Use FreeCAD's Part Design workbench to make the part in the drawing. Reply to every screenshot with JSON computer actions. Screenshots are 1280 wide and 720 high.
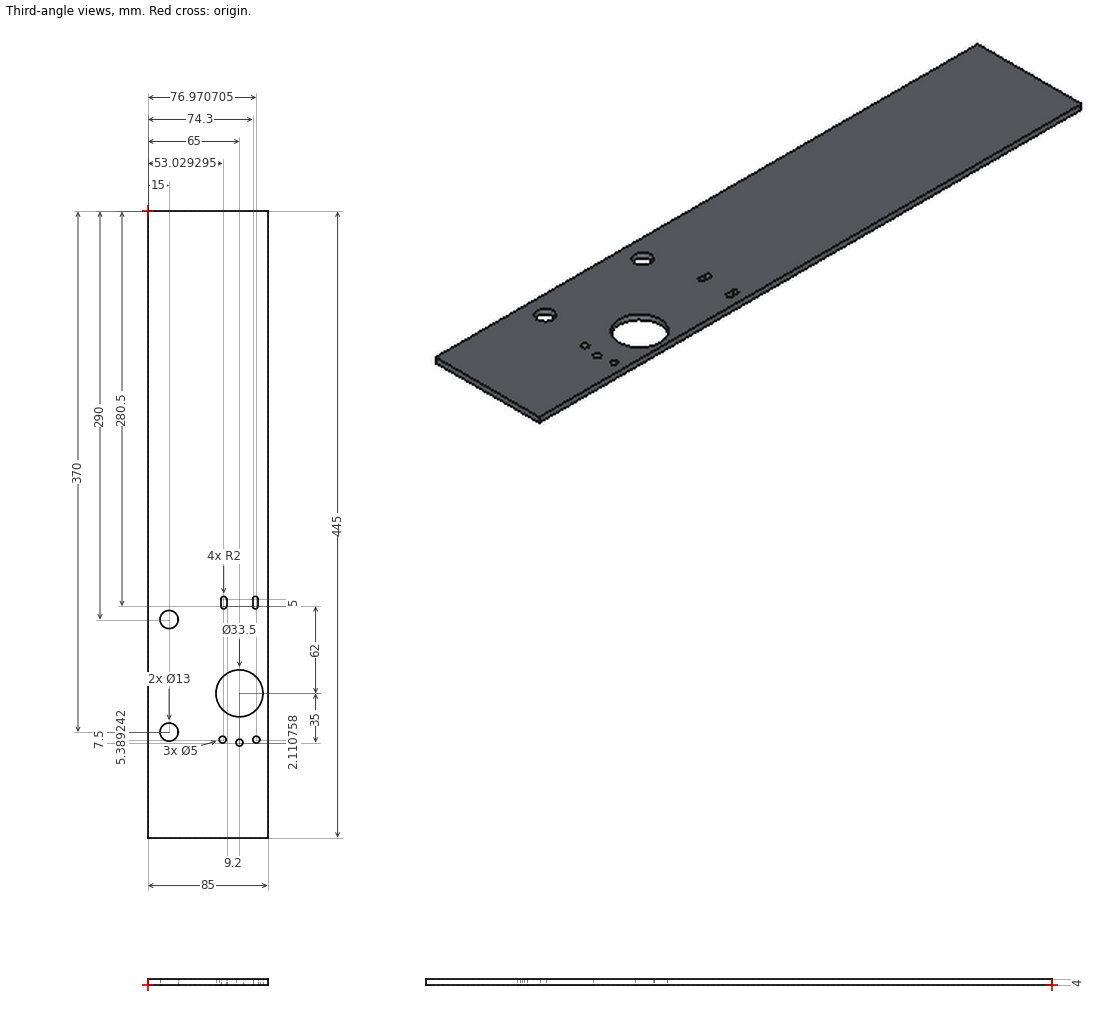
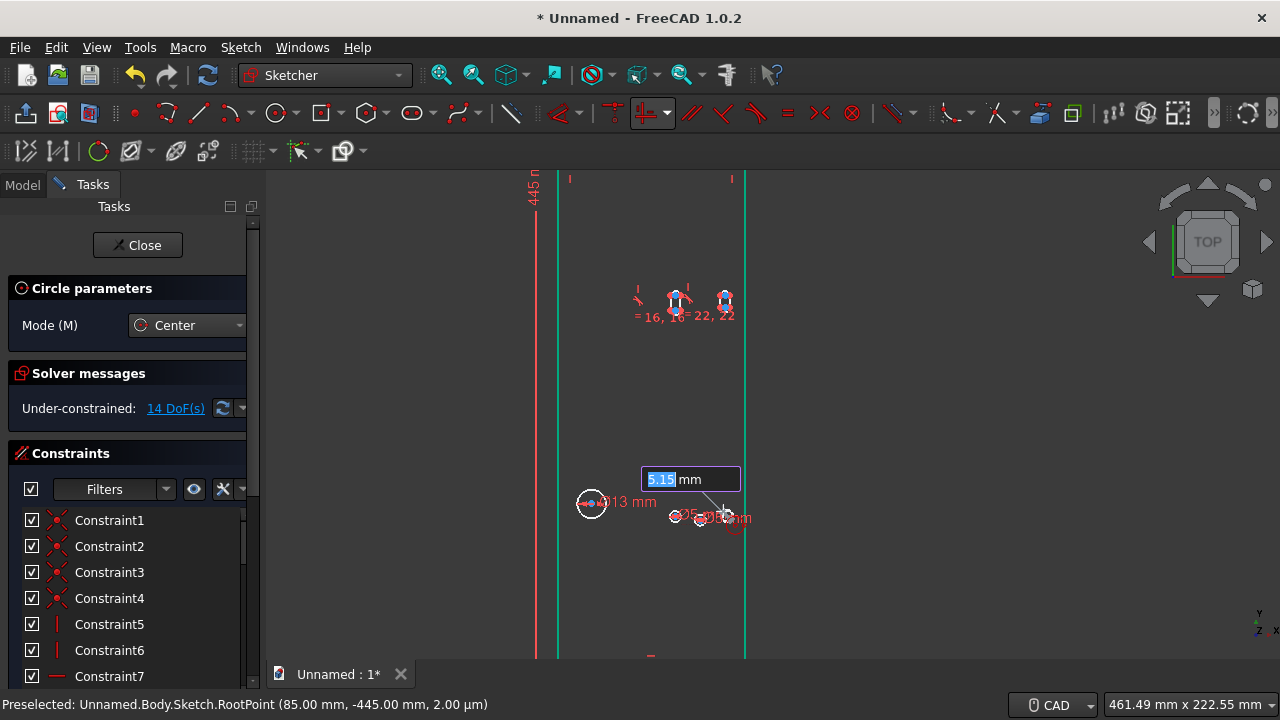
{"action": "type", "text": "5"}
{"action": "key", "text": "Return"}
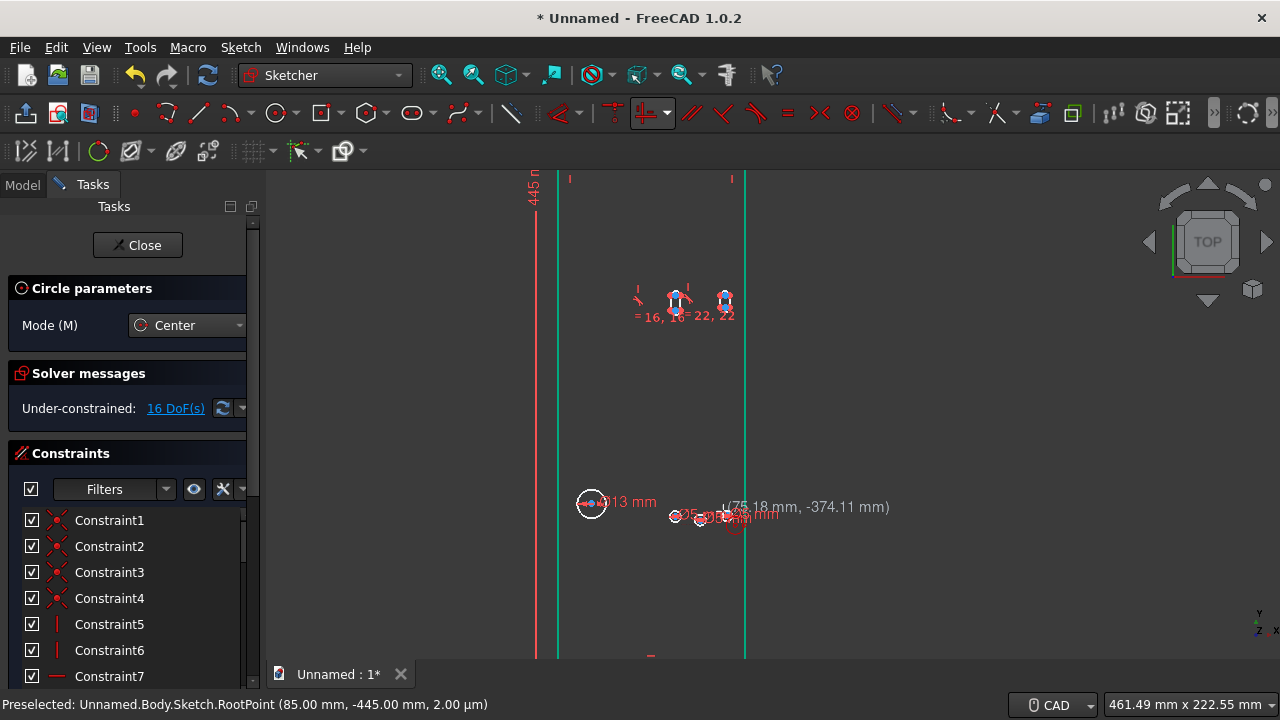
{"action": "left_click", "coordinate": [701, 443]}
{"action": "mouse_move", "coordinate": [727, 417]}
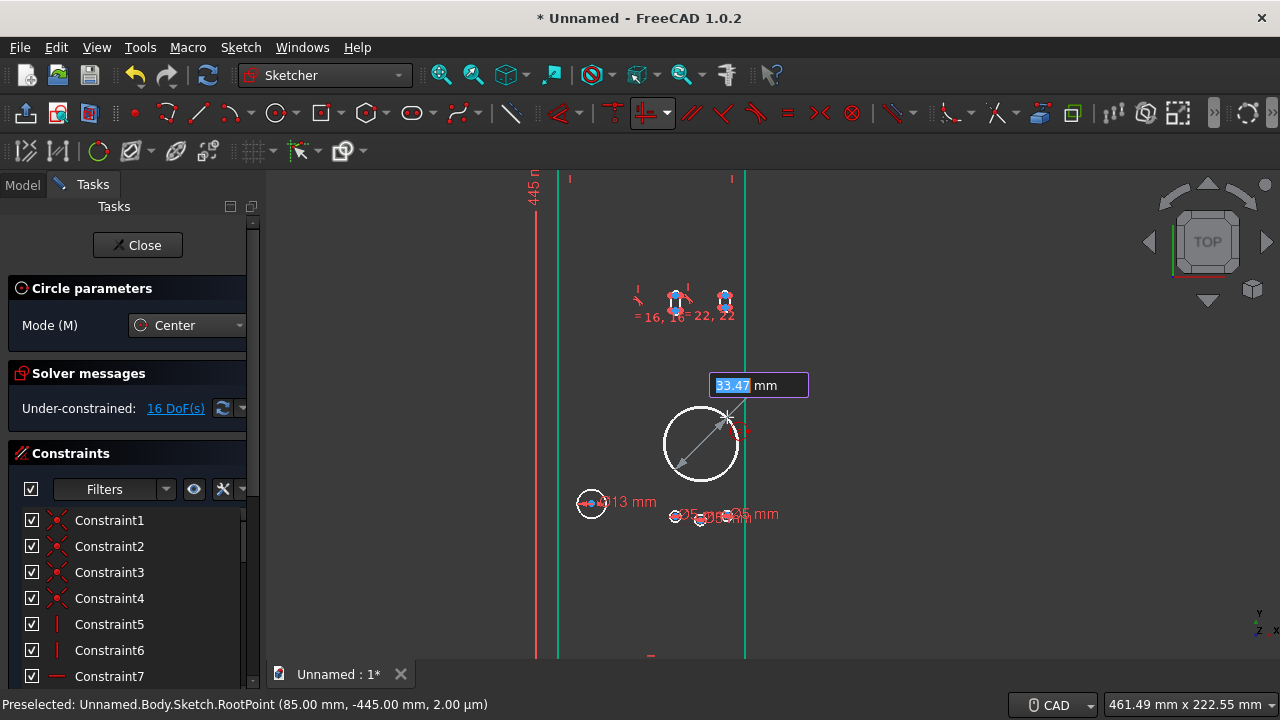
{"action": "type", "text": "33.5"}
{"action": "key", "text": "Return"}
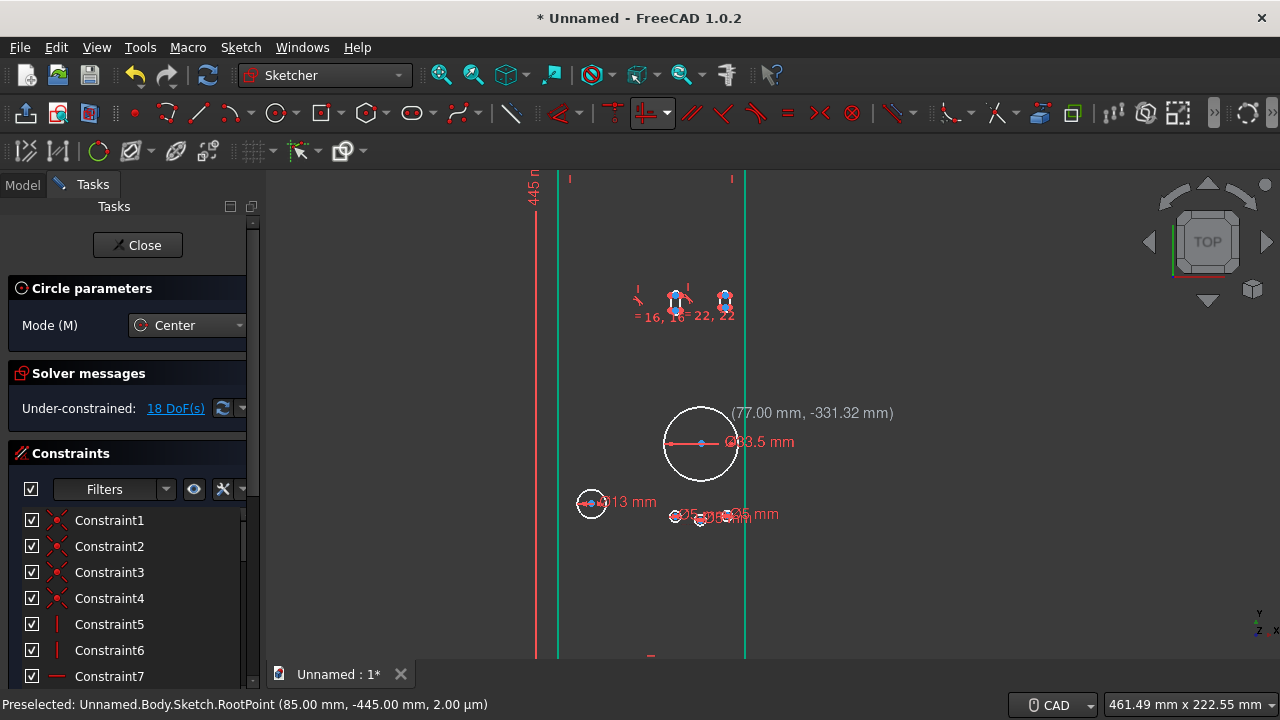
{"action": "scroll", "coordinate": [591, 327], "scroll_direction": "up", "scroll_amount": 3}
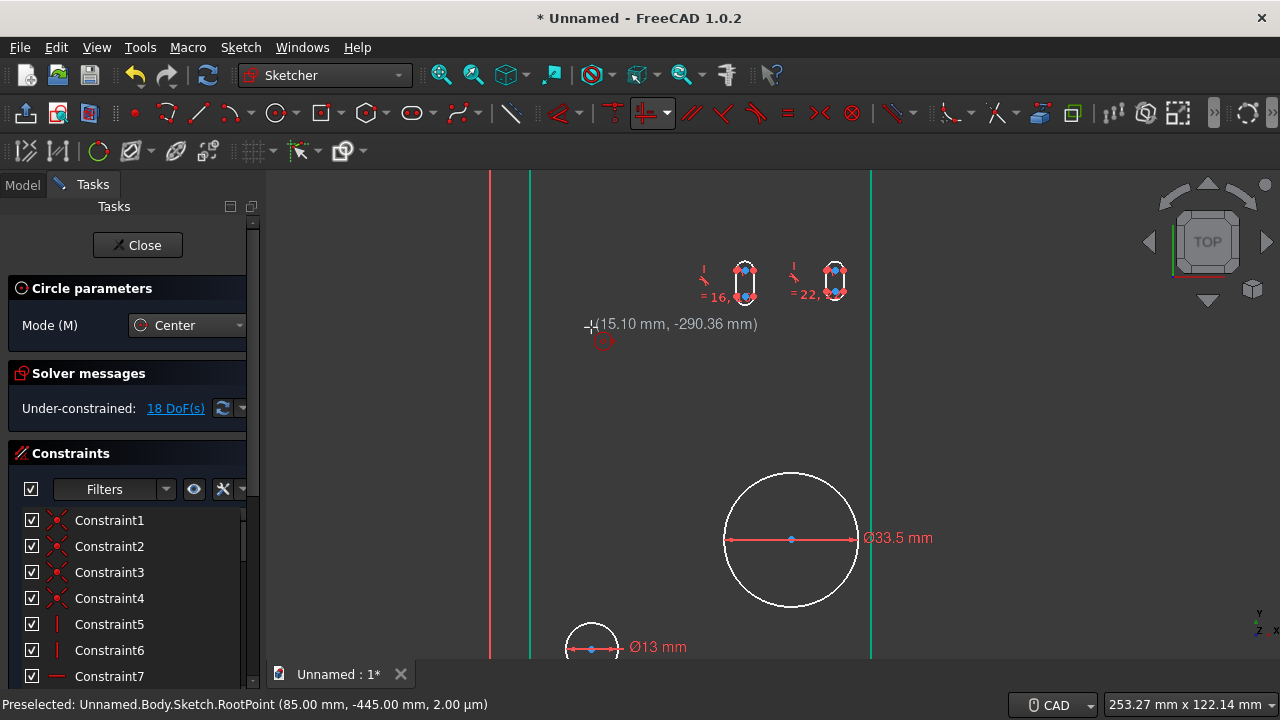
{"action": "scroll", "coordinate": [705, 485], "scroll_direction": "down", "scroll_amount": 9}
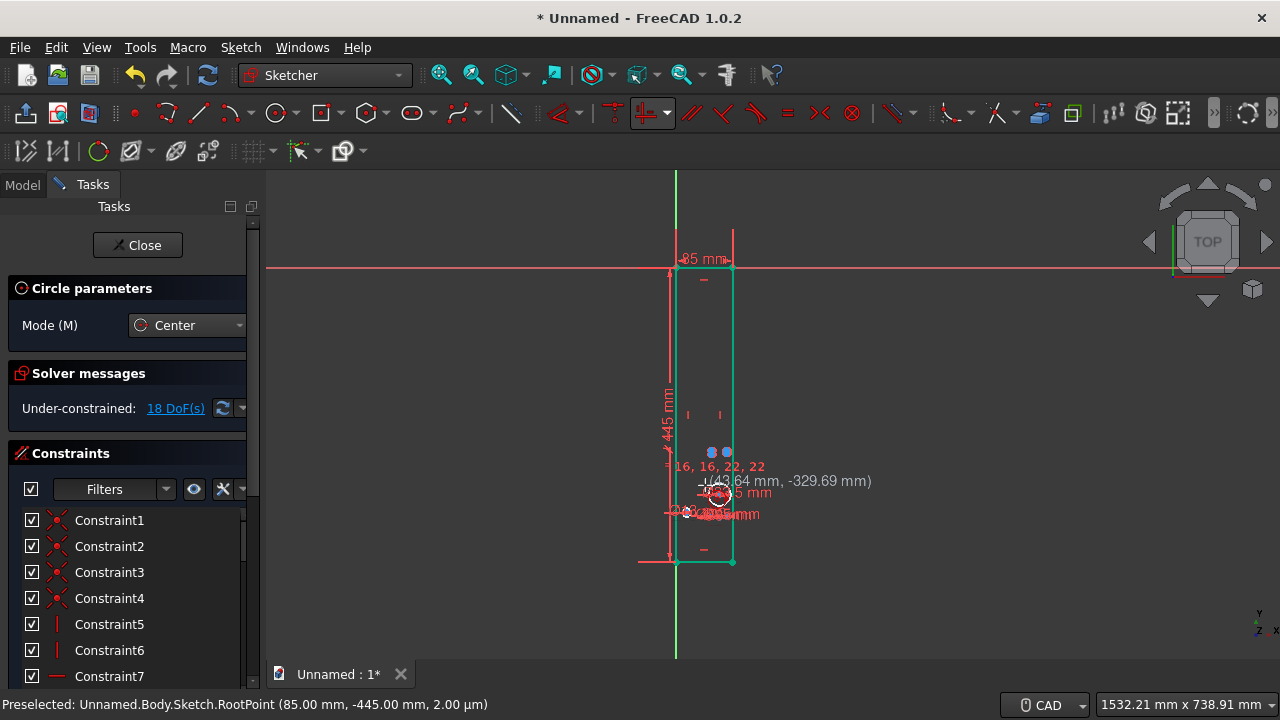
{"action": "scroll", "coordinate": [686, 459], "scroll_direction": "up", "scroll_amount": 3}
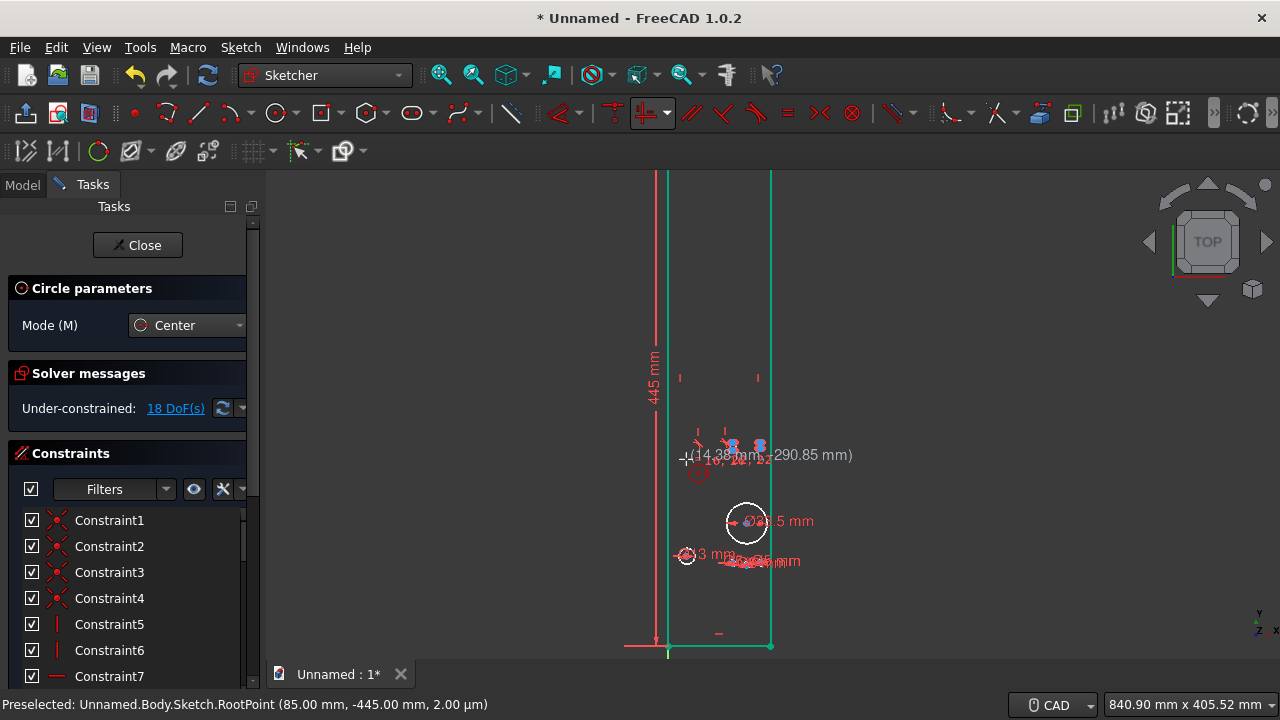
{"action": "left_click", "coordinate": [686, 459]}
{"action": "mouse_move", "coordinate": [692, 454]}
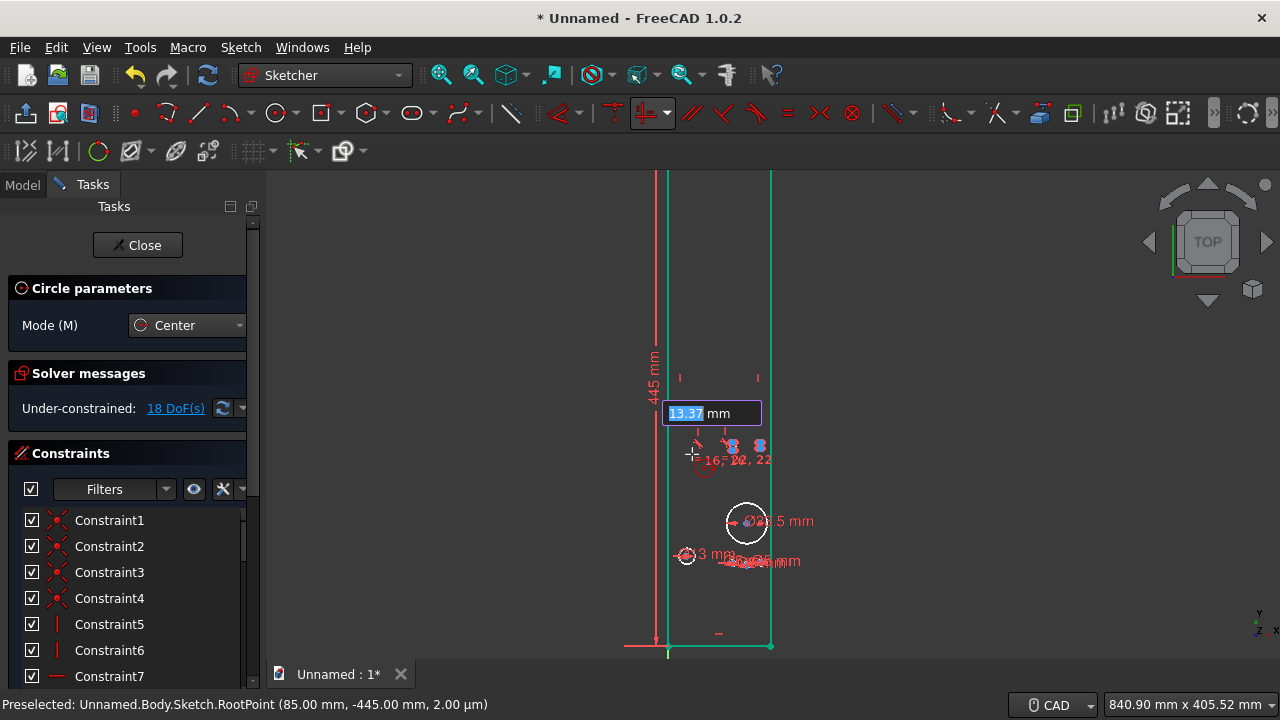
{"action": "type", "text": "13"}
{"action": "key", "text": "Return"}
{"action": "key", "text": "Escape"}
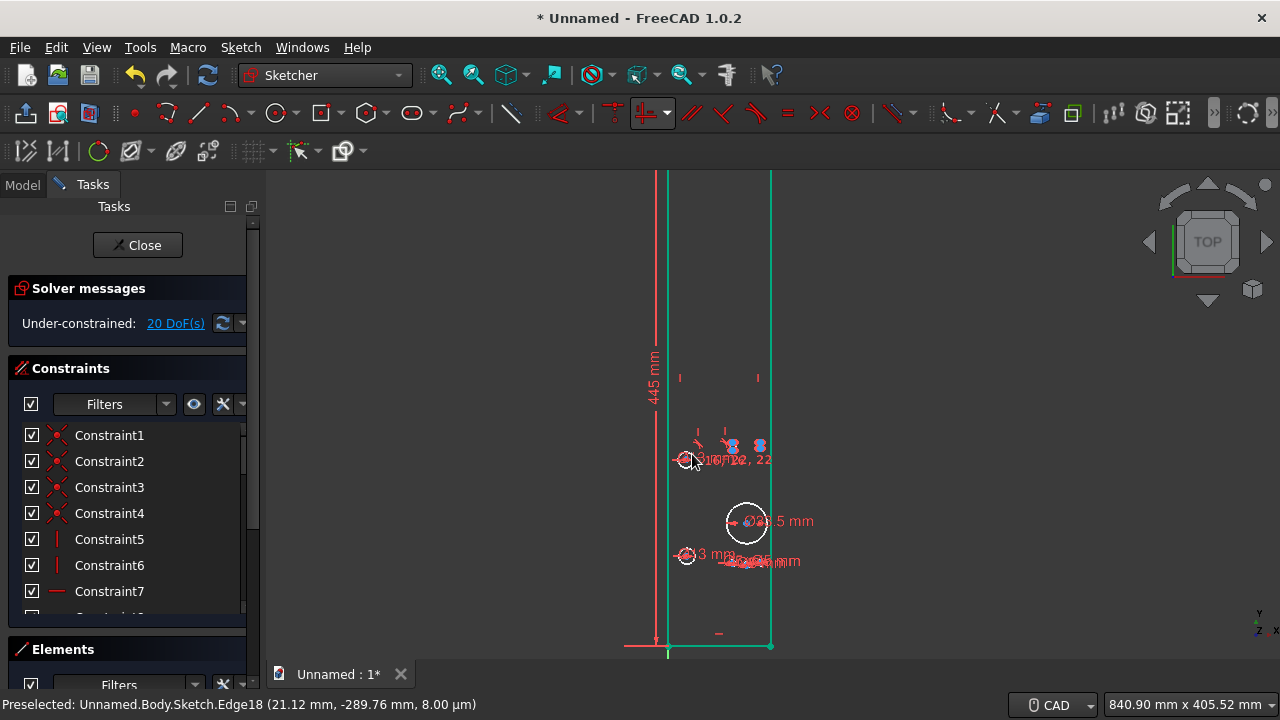
{"action": "scroll", "coordinate": [733, 453], "scroll_direction": "up", "scroll_amount": 9}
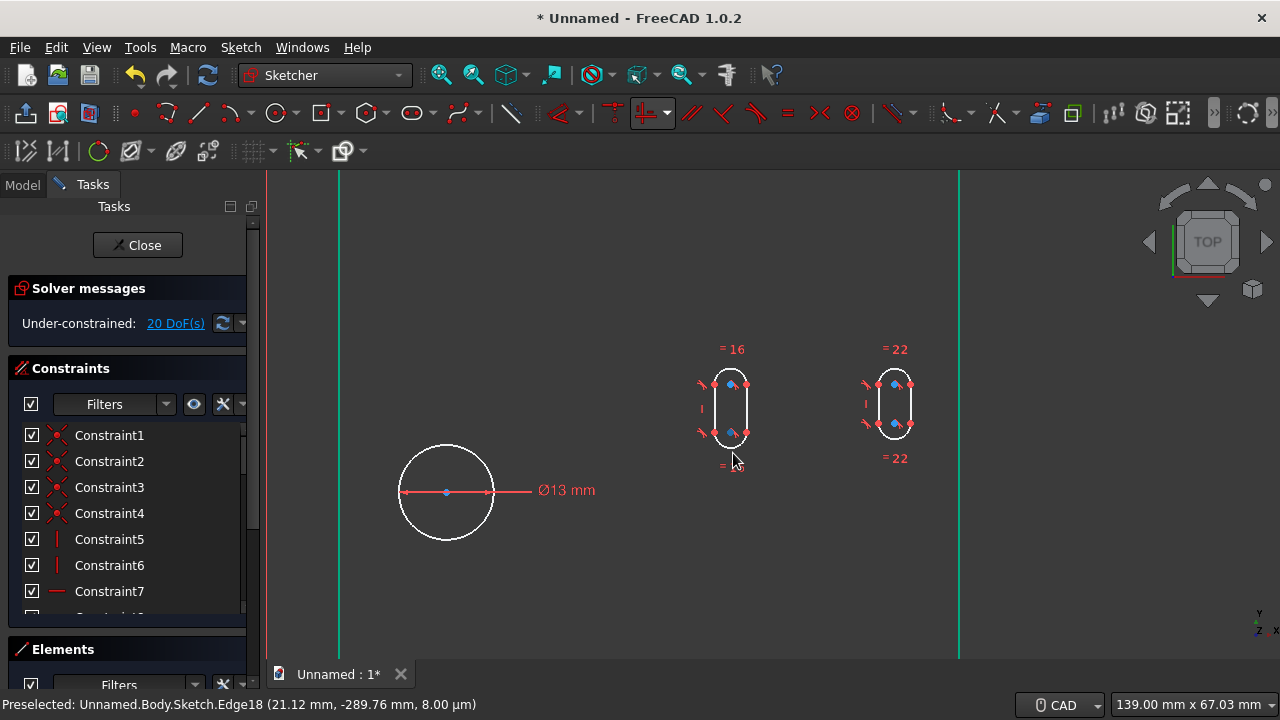
{"action": "left_click", "coordinate": [731, 448]}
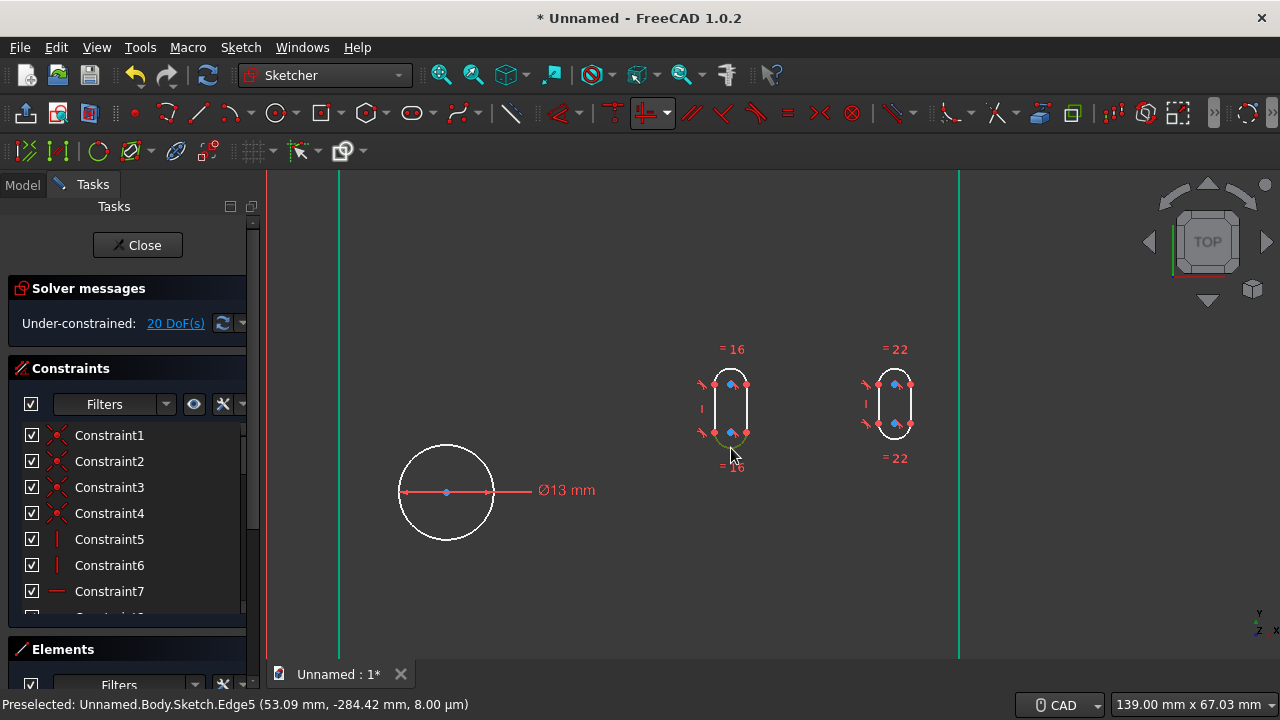
{"action": "left_click", "coordinate": [885, 436]}